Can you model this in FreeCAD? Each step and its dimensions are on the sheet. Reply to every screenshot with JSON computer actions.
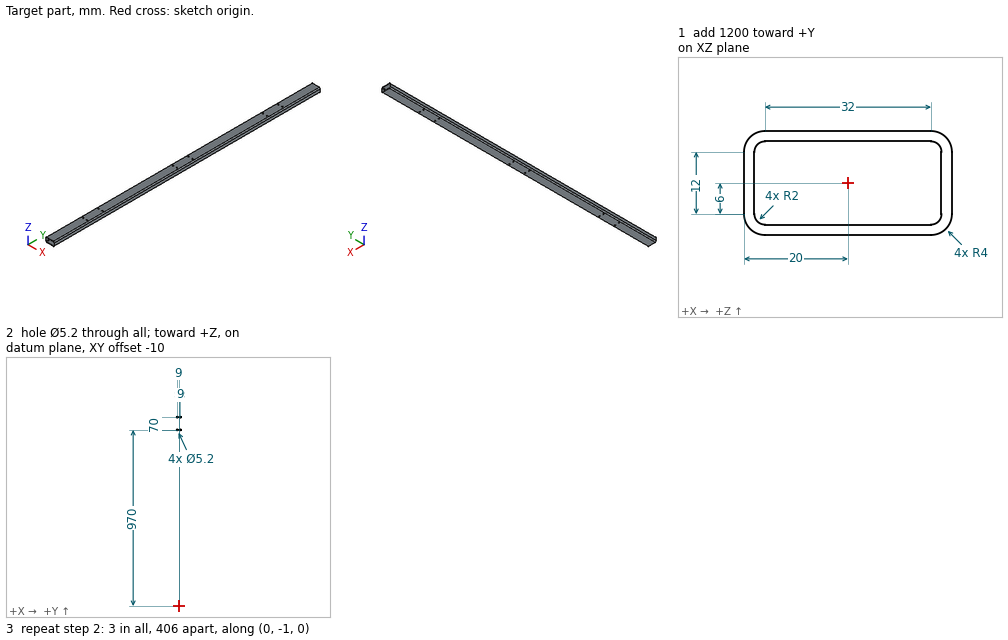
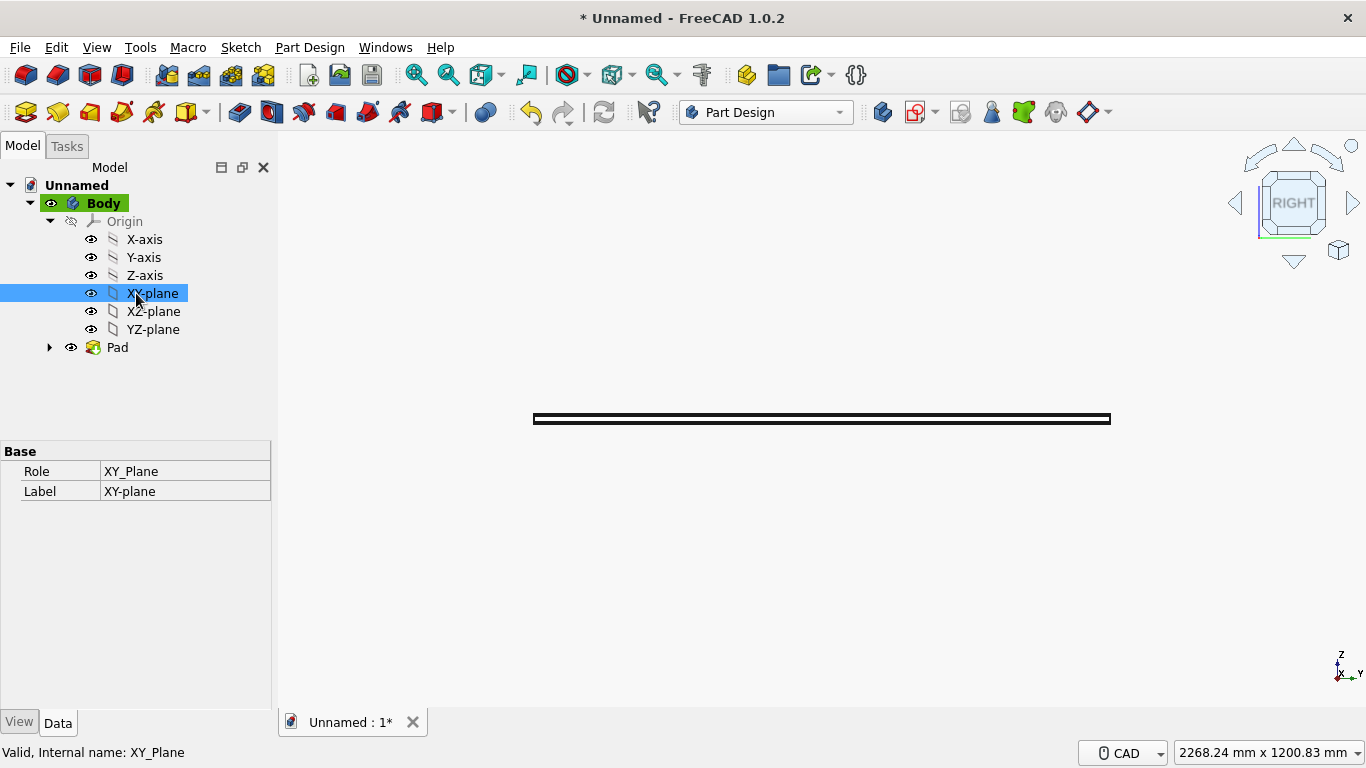
{"action": "left_click", "coordinate": [1088, 112]}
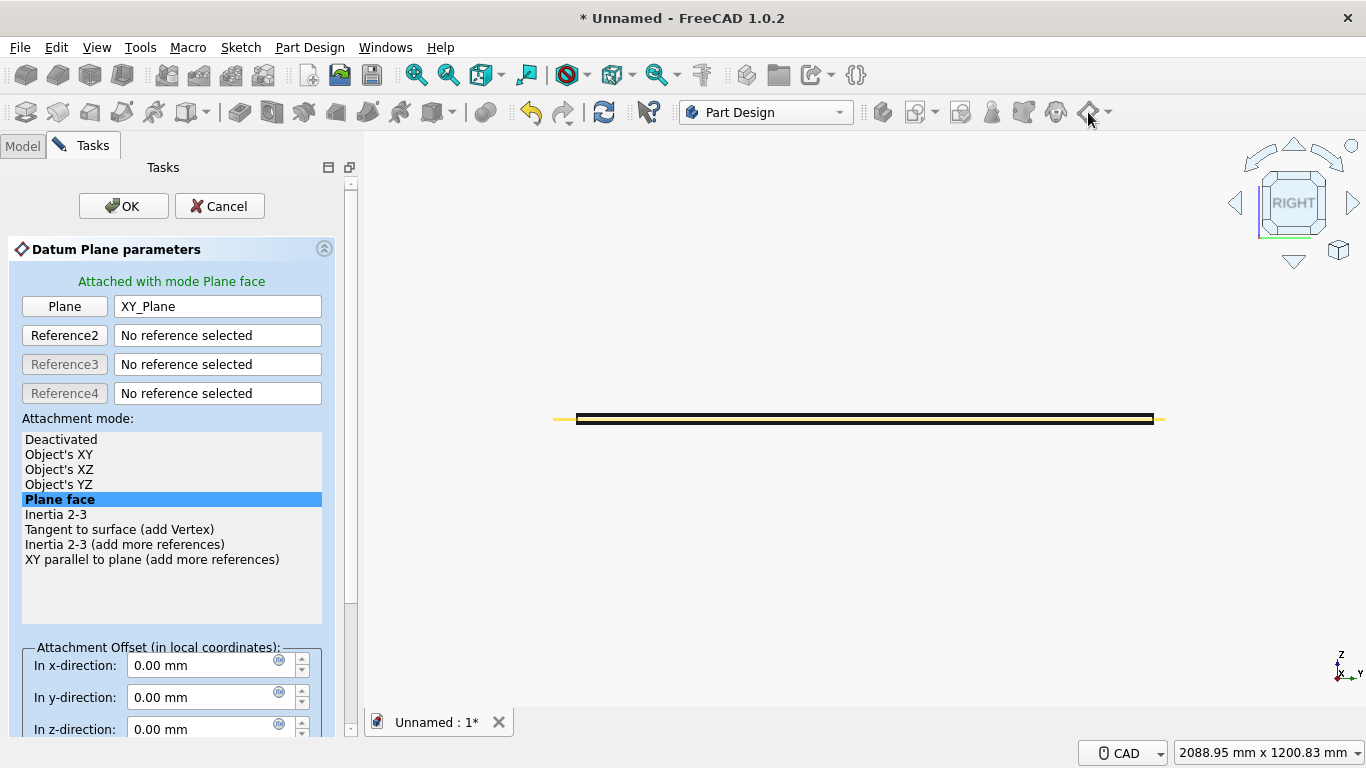
{"action": "scroll", "coordinate": [351, 456], "scroll_direction": "down", "scroll_amount": 2}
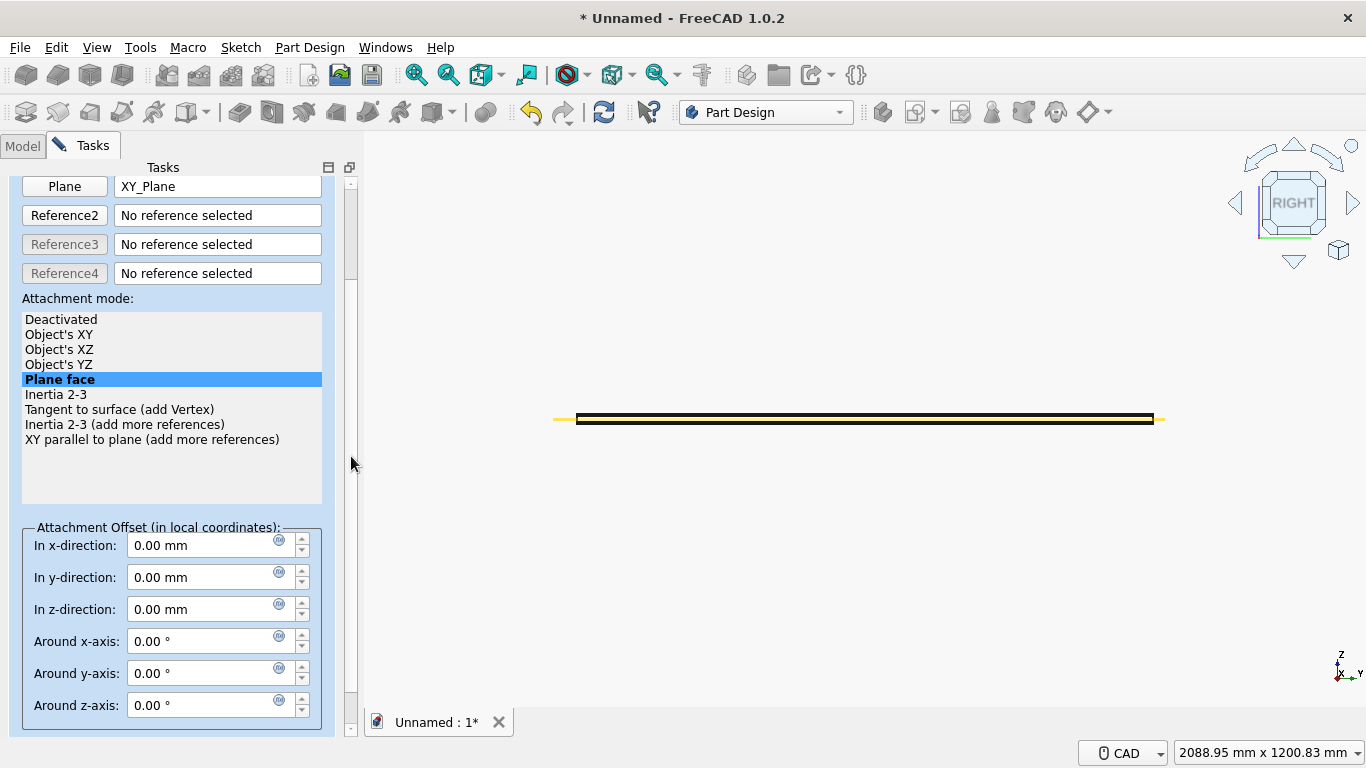
{"action": "triple_click", "coordinate": [210, 609]}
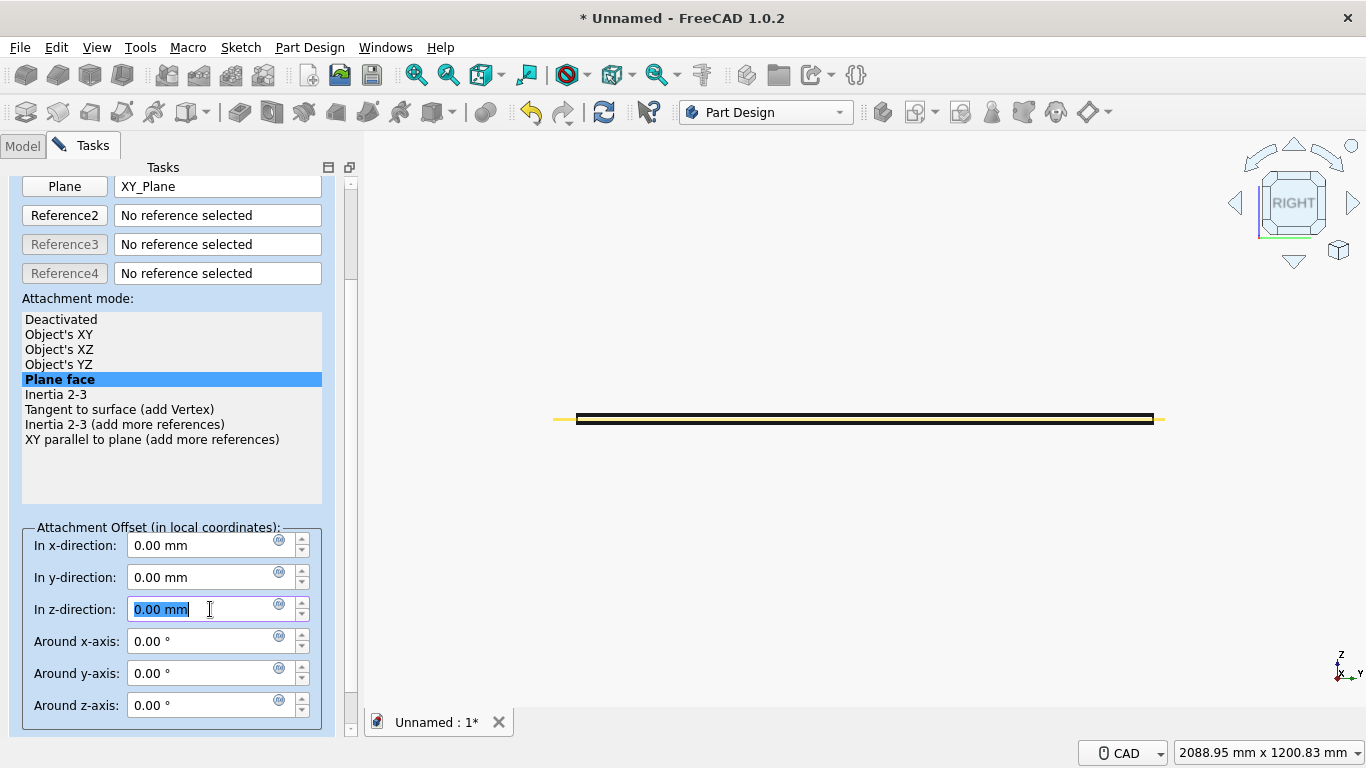
{"action": "type", "text": "-10"}
{"action": "key", "text": "Tab"}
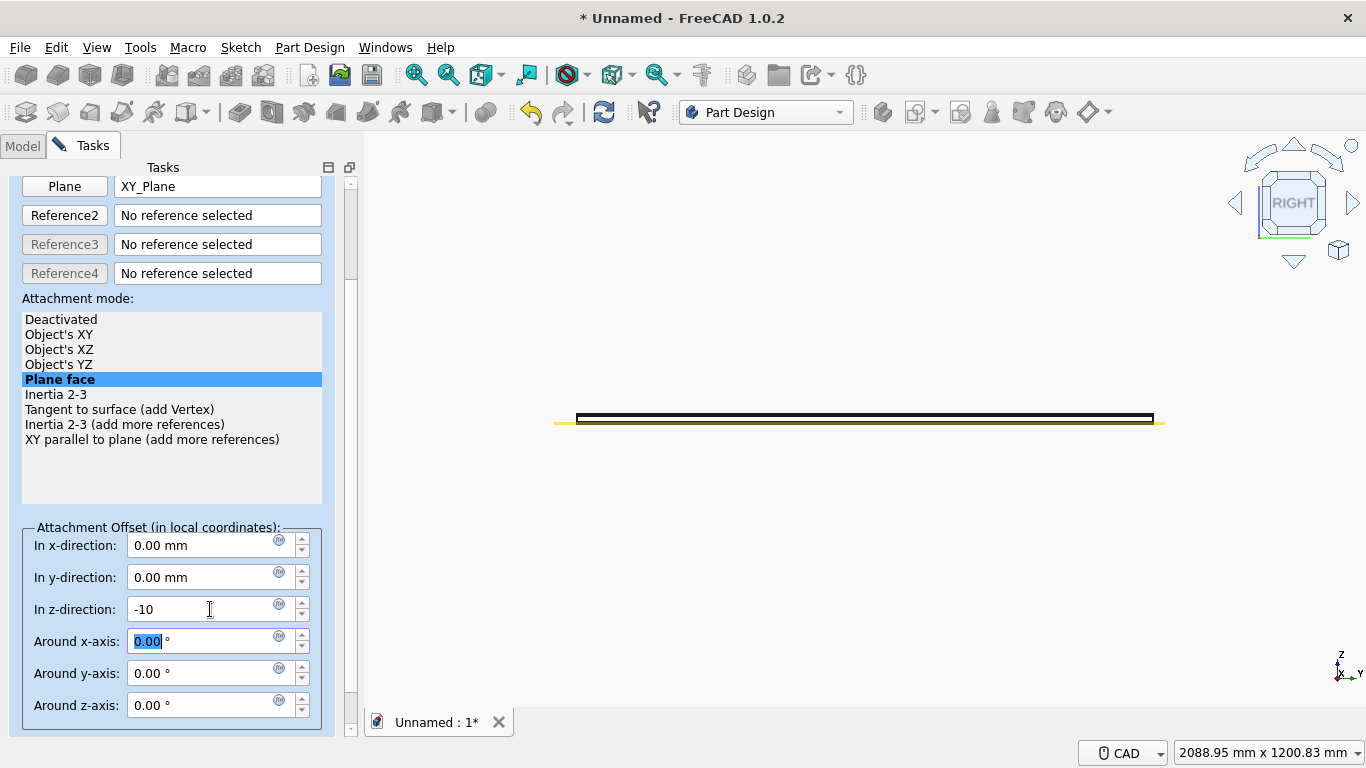
{"action": "scroll", "coordinate": [351, 456], "scroll_direction": "up", "scroll_amount": 3}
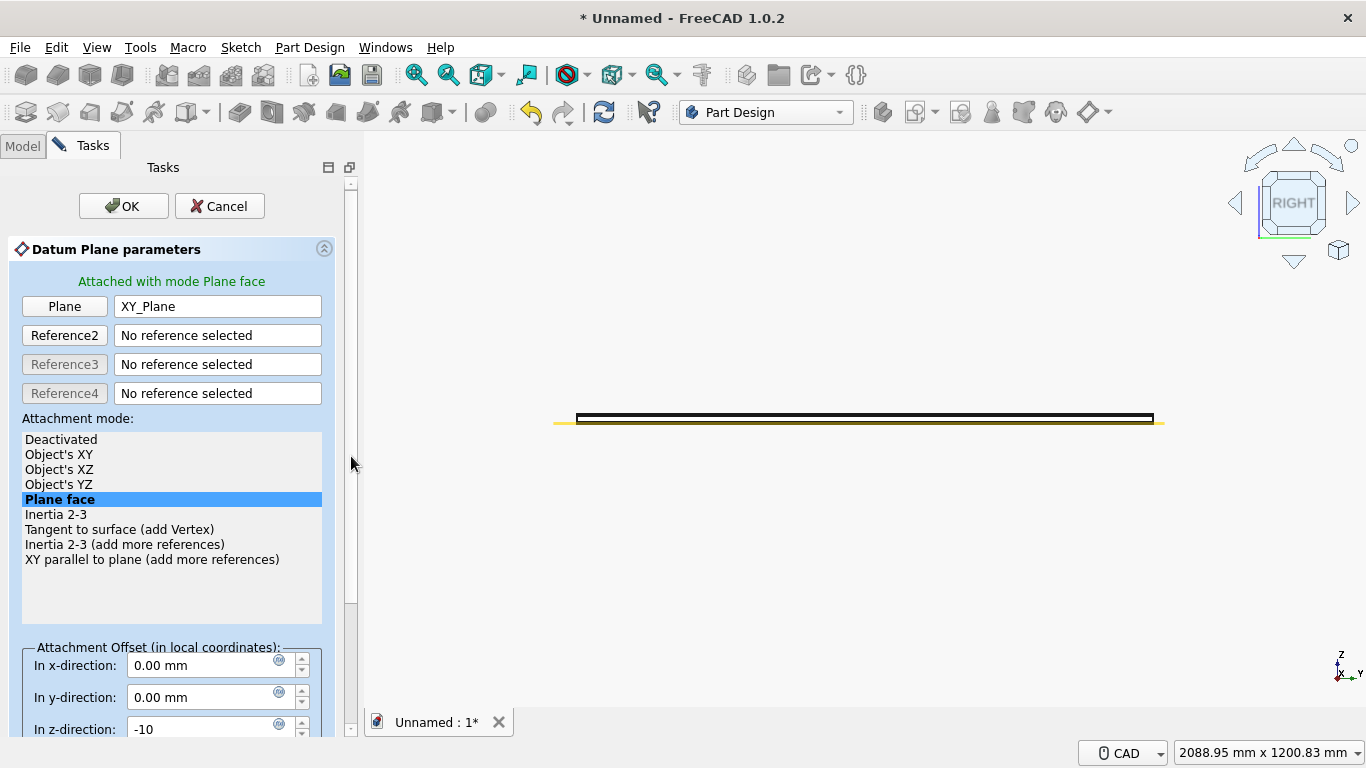
{"action": "left_click", "coordinate": [124, 206]}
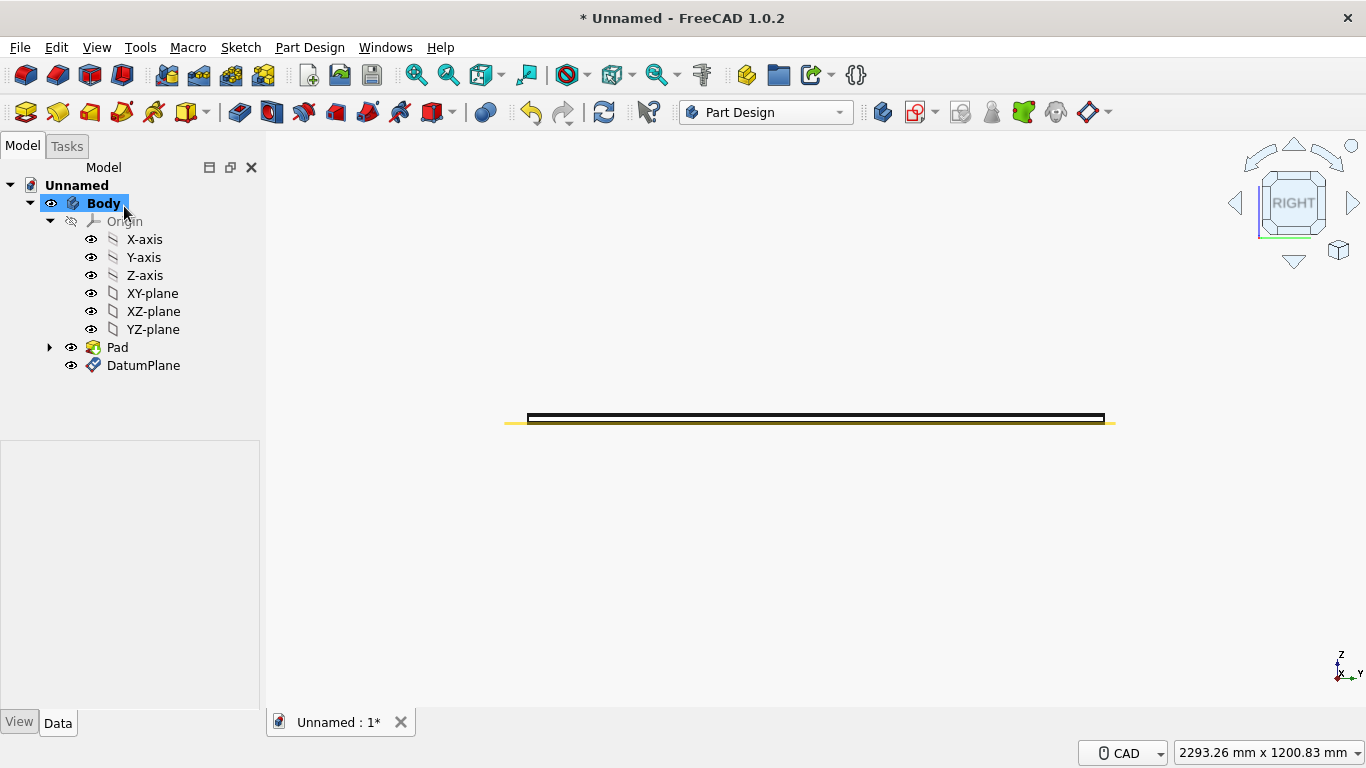
{"action": "left_click", "coordinate": [116, 365]}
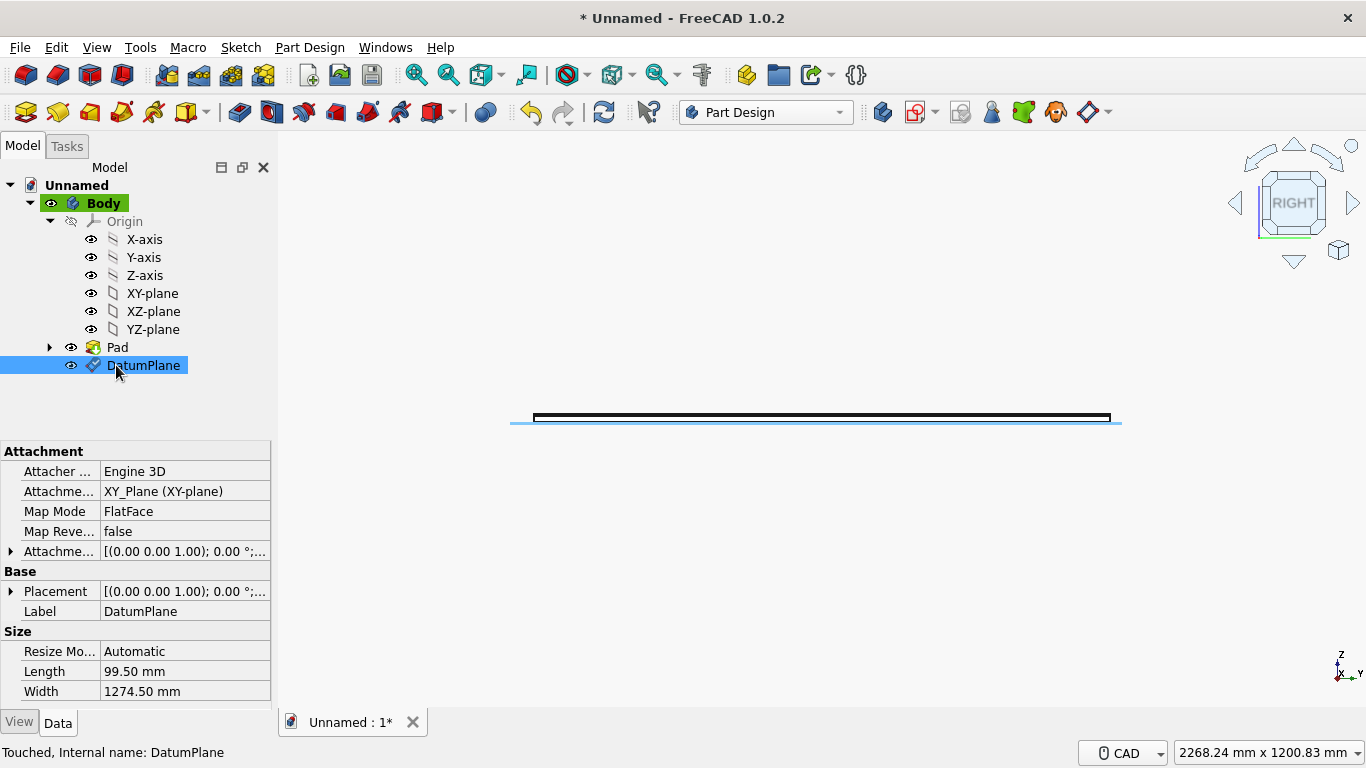
{"action": "left_click", "coordinate": [916, 112]}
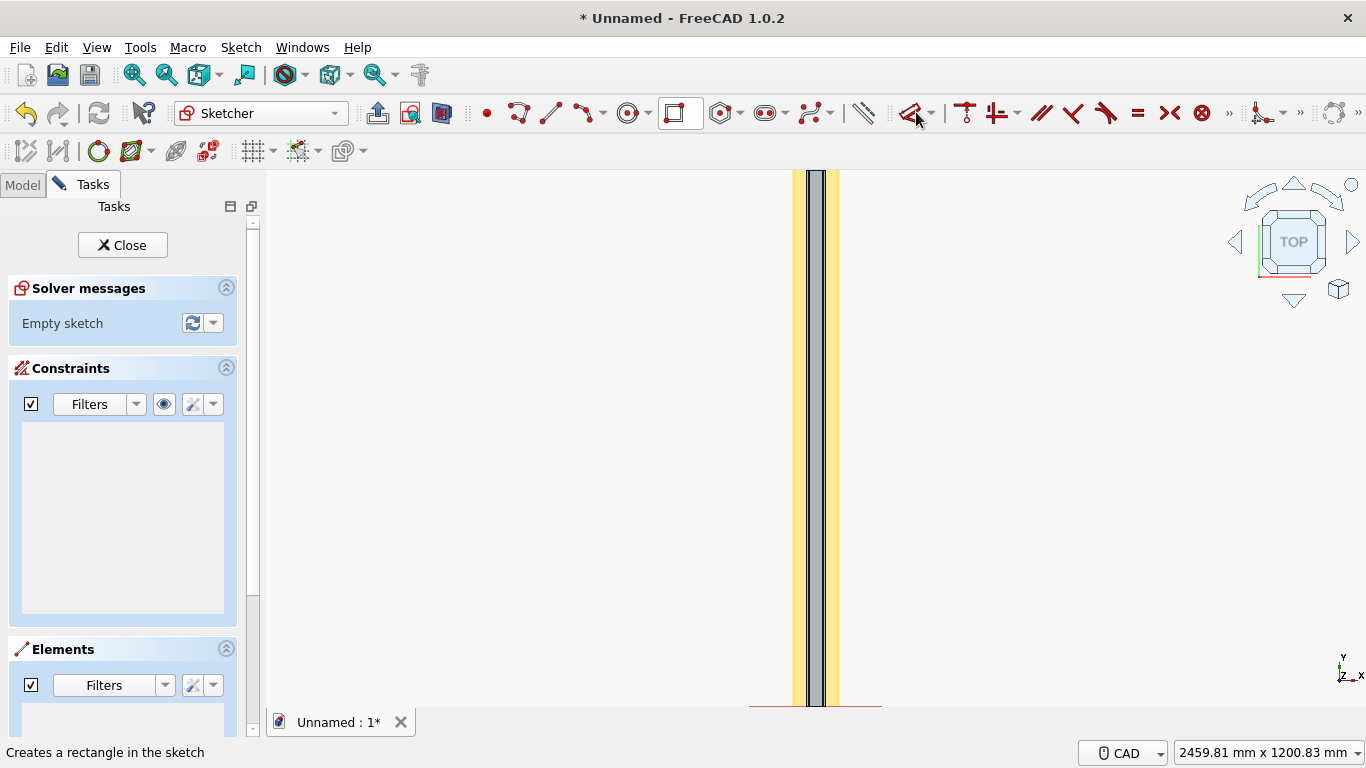
{"action": "left_click", "coordinate": [442, 114]}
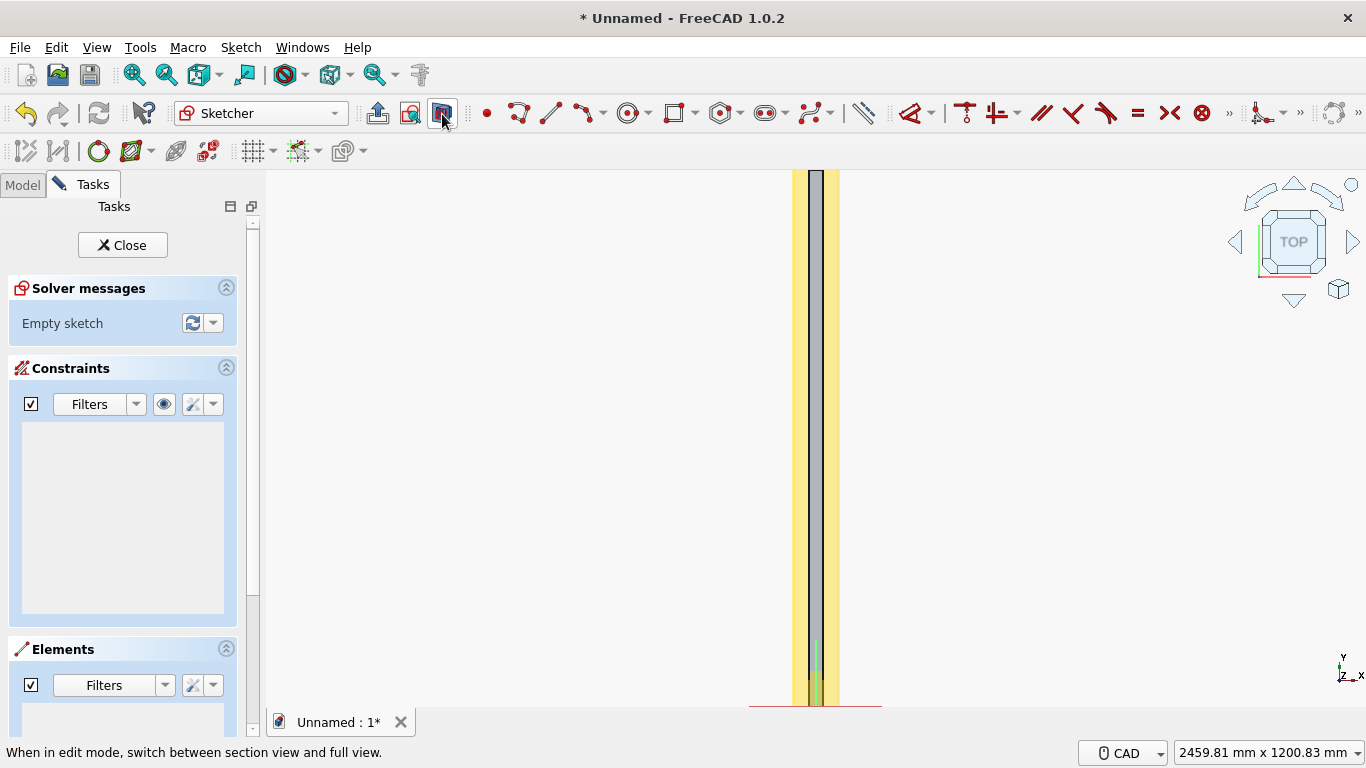
{"action": "scroll", "coordinate": [823, 239], "scroll_direction": "up", "scroll_amount": 12}